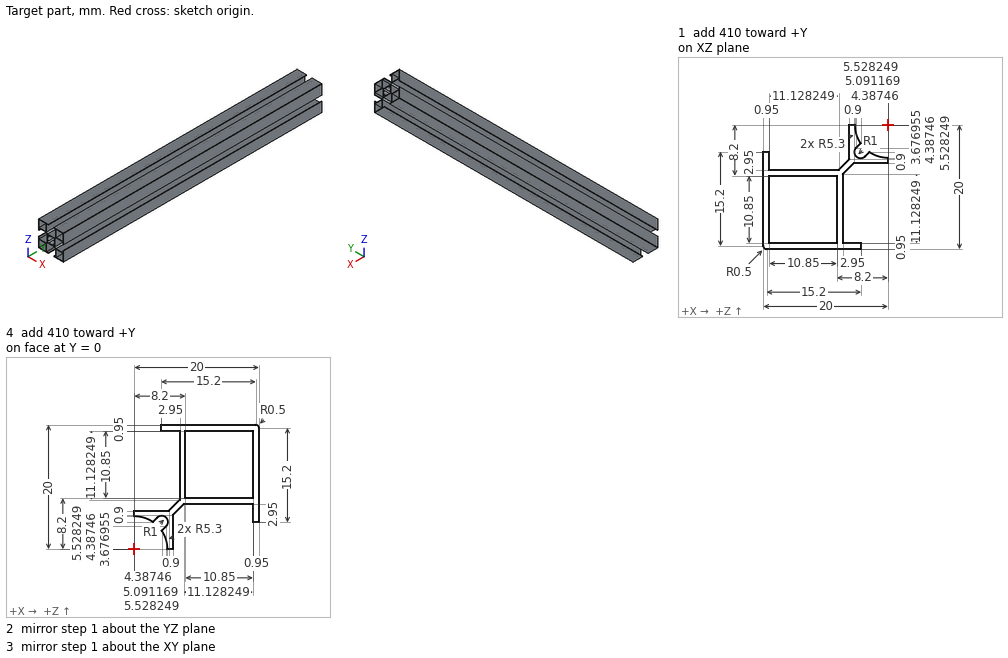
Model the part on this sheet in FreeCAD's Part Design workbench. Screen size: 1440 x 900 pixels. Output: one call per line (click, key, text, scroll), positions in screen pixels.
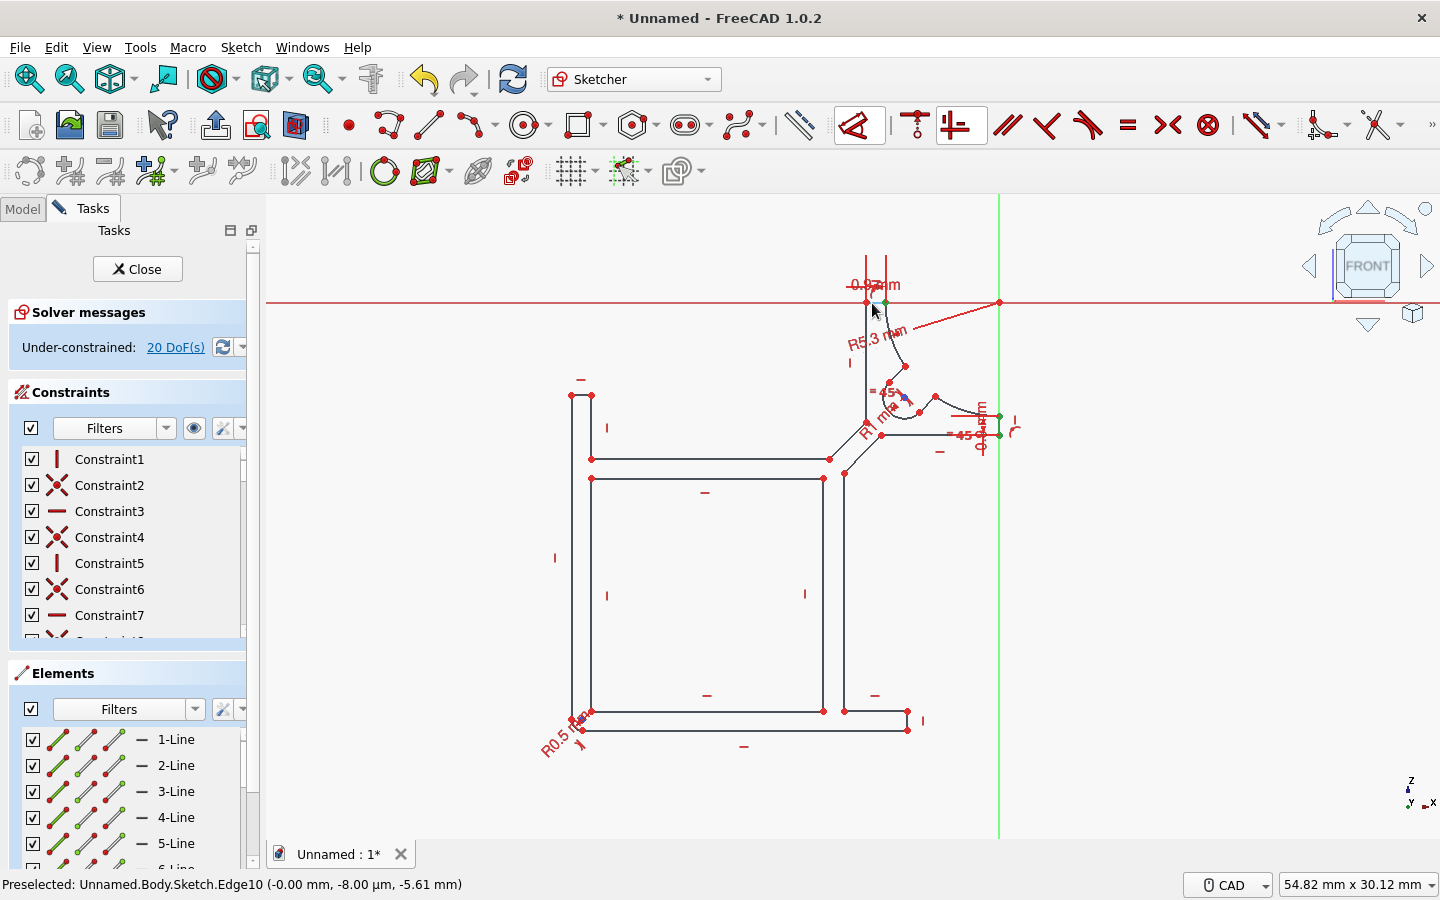
click(572, 720)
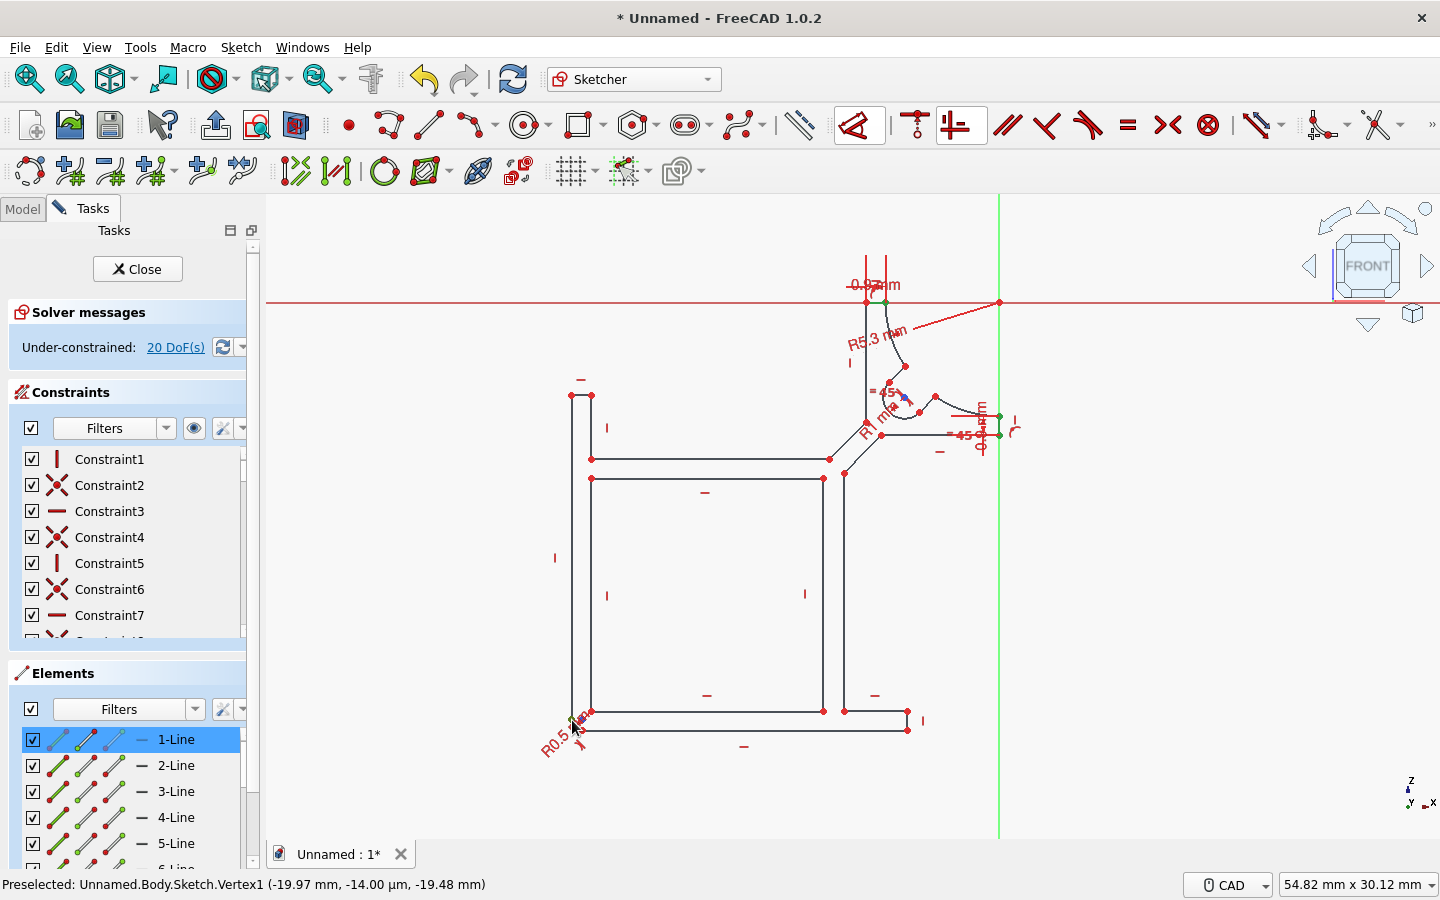
key(l)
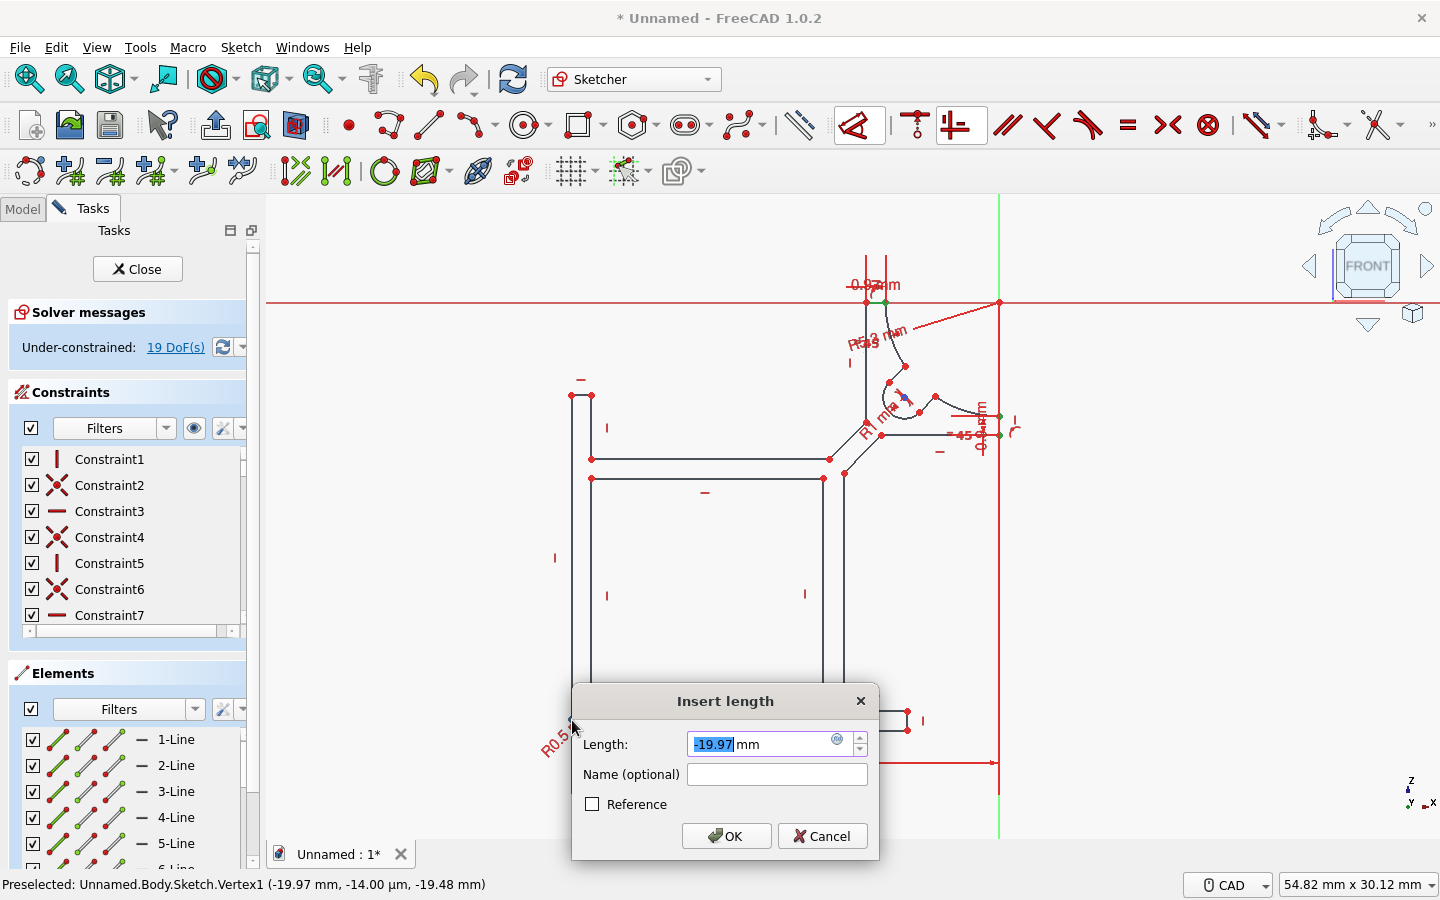
text(-20)
key(Return)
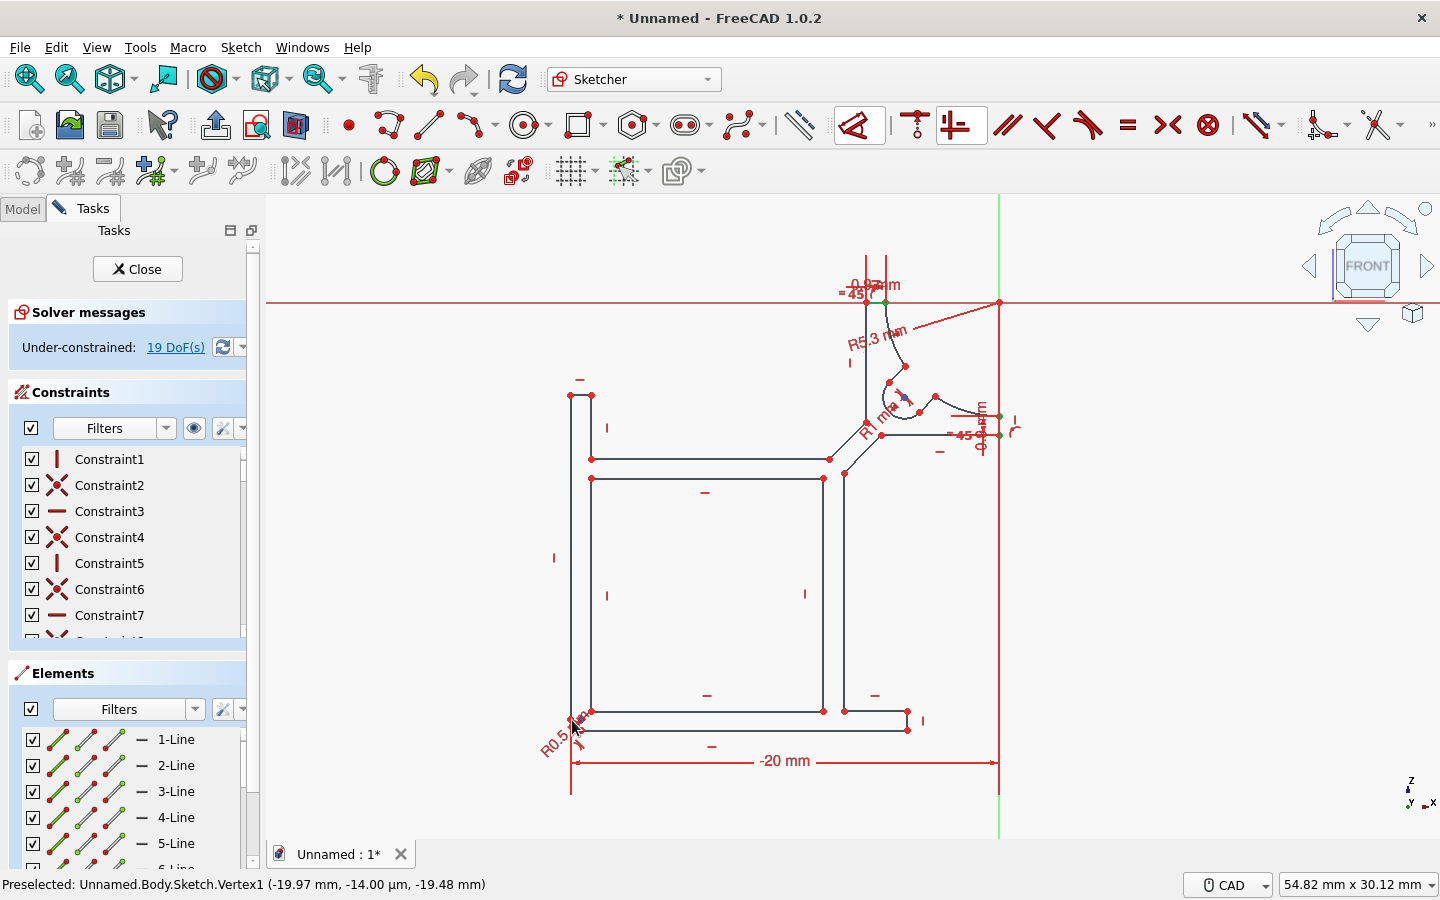
click(907, 731)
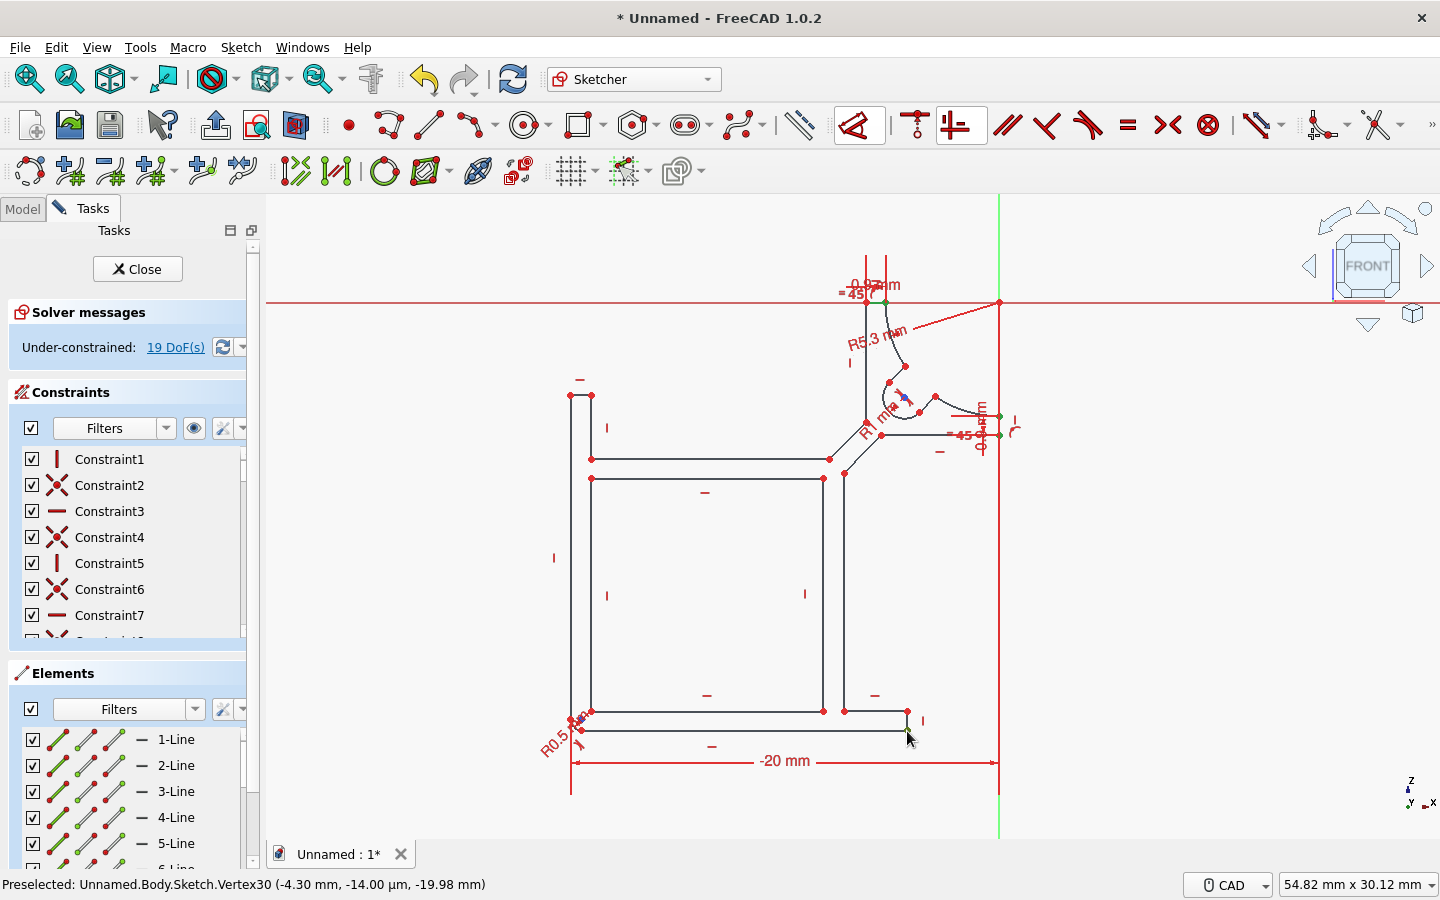
key(i)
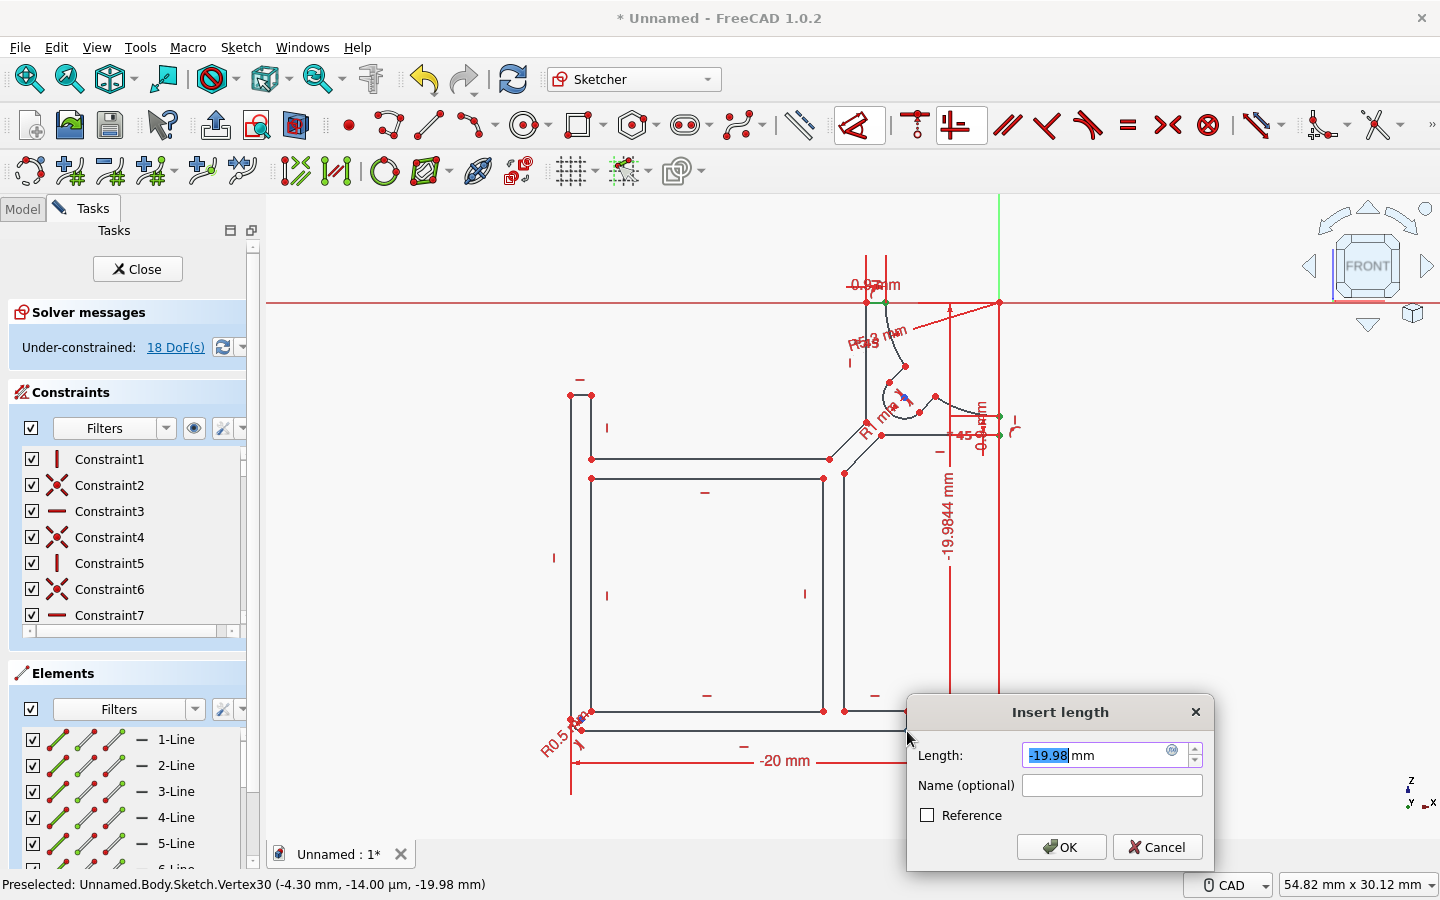
text(-20)
key(Return)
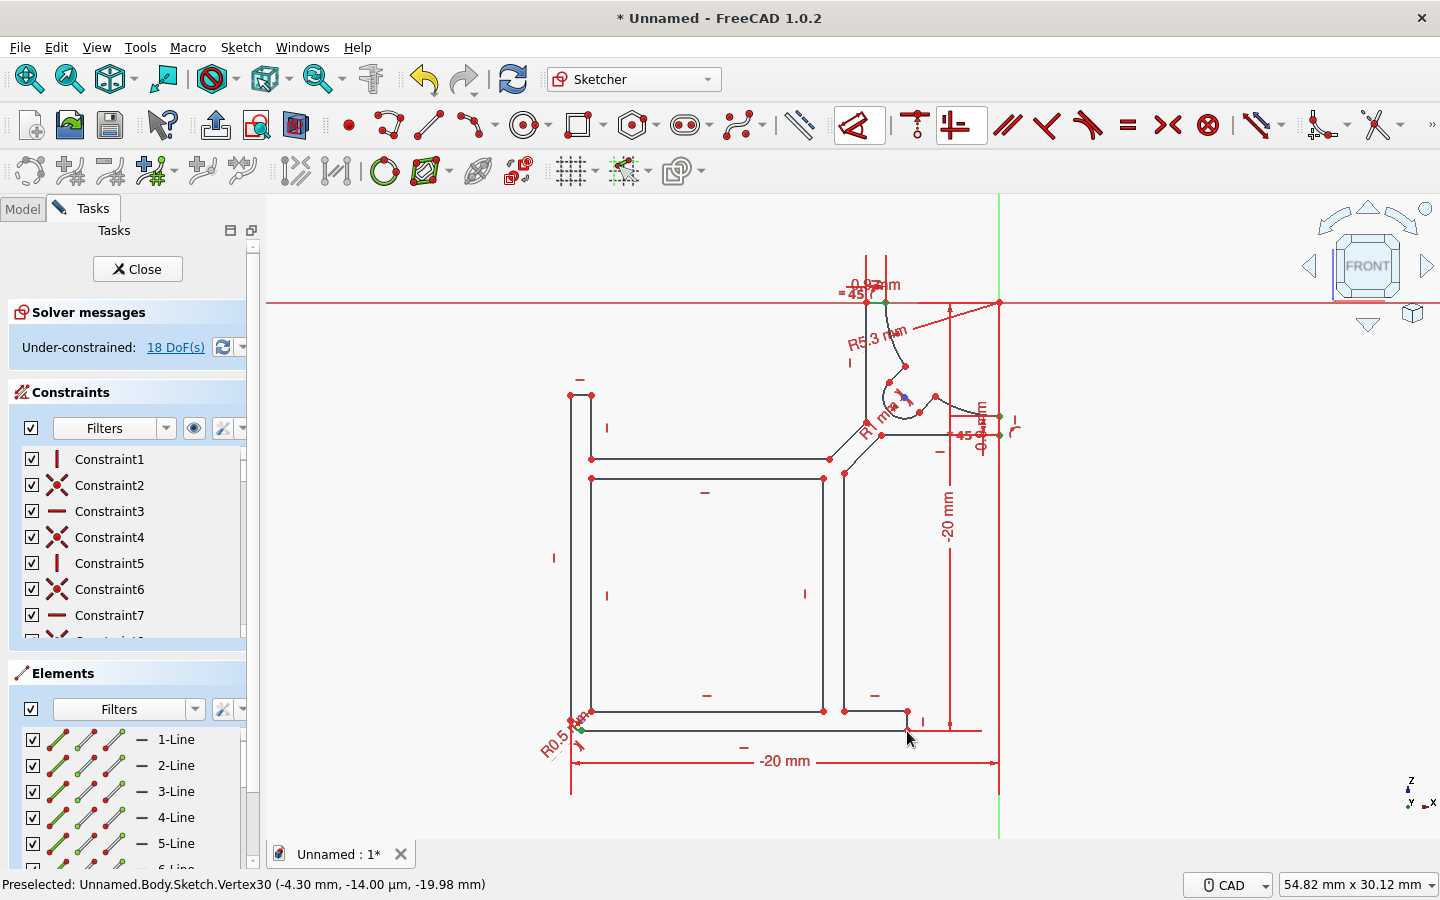
click(571, 623)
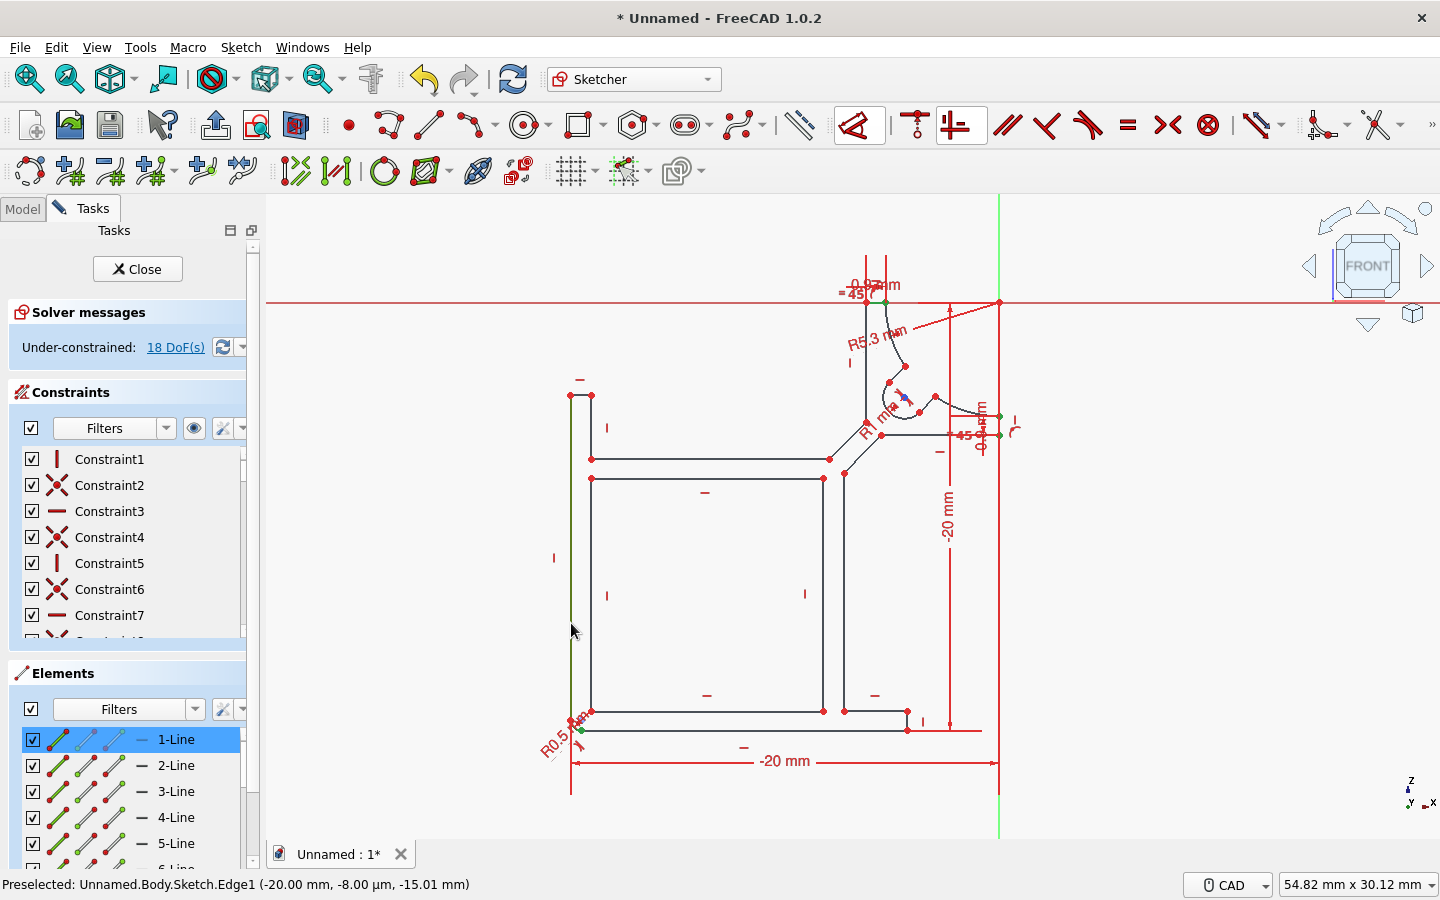
click(880, 126)